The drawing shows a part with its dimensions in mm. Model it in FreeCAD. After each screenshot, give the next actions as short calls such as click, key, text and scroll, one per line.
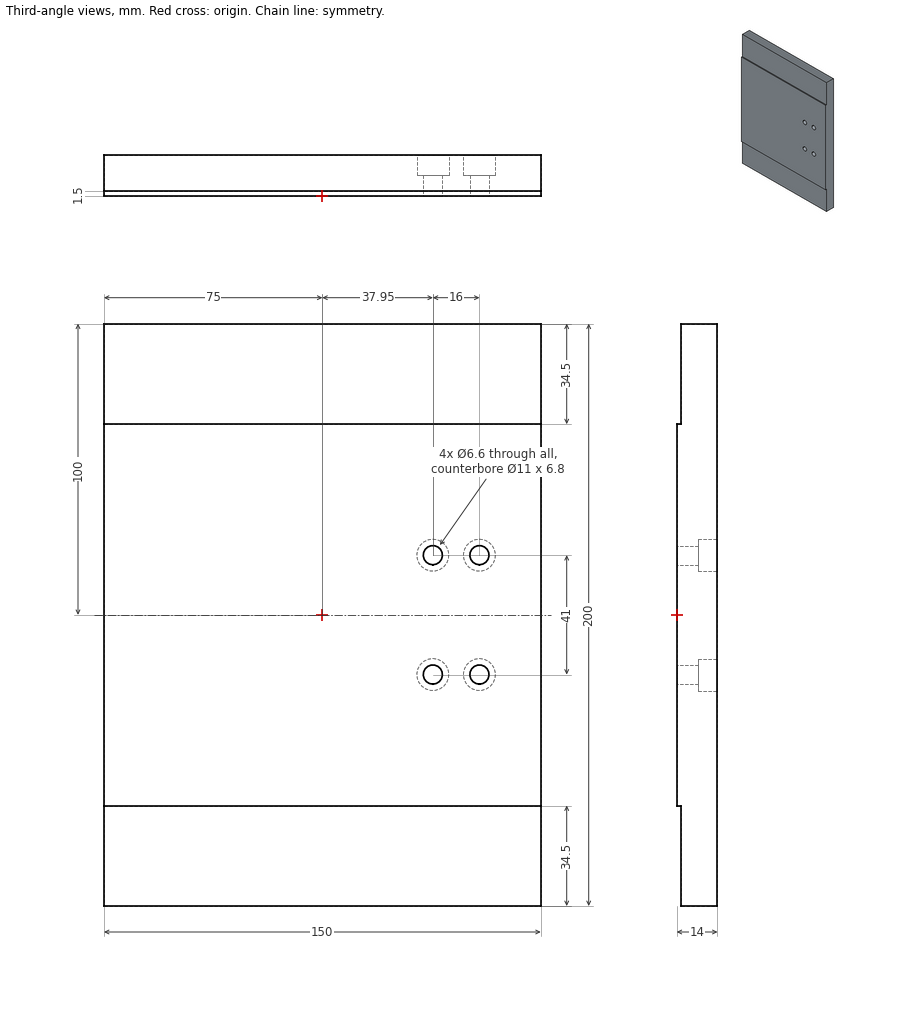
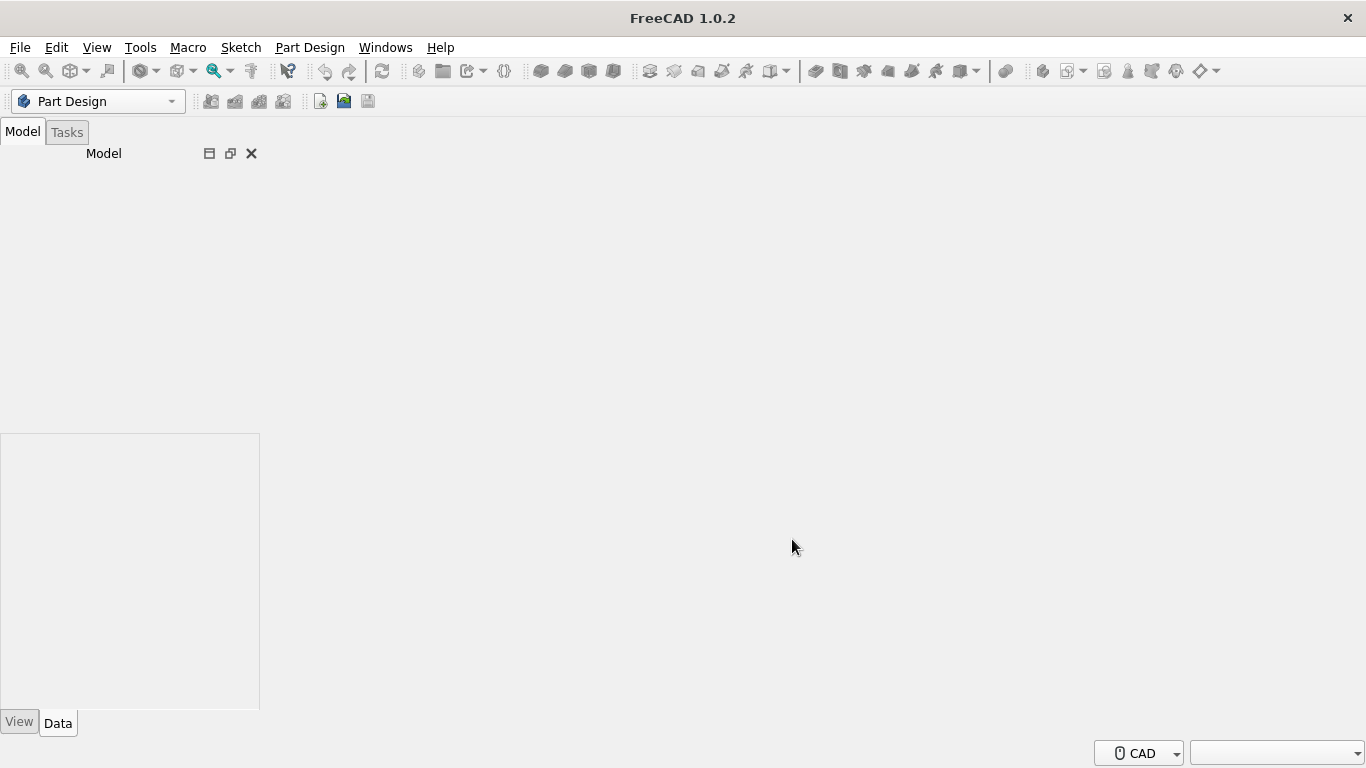
key(ctrl+n)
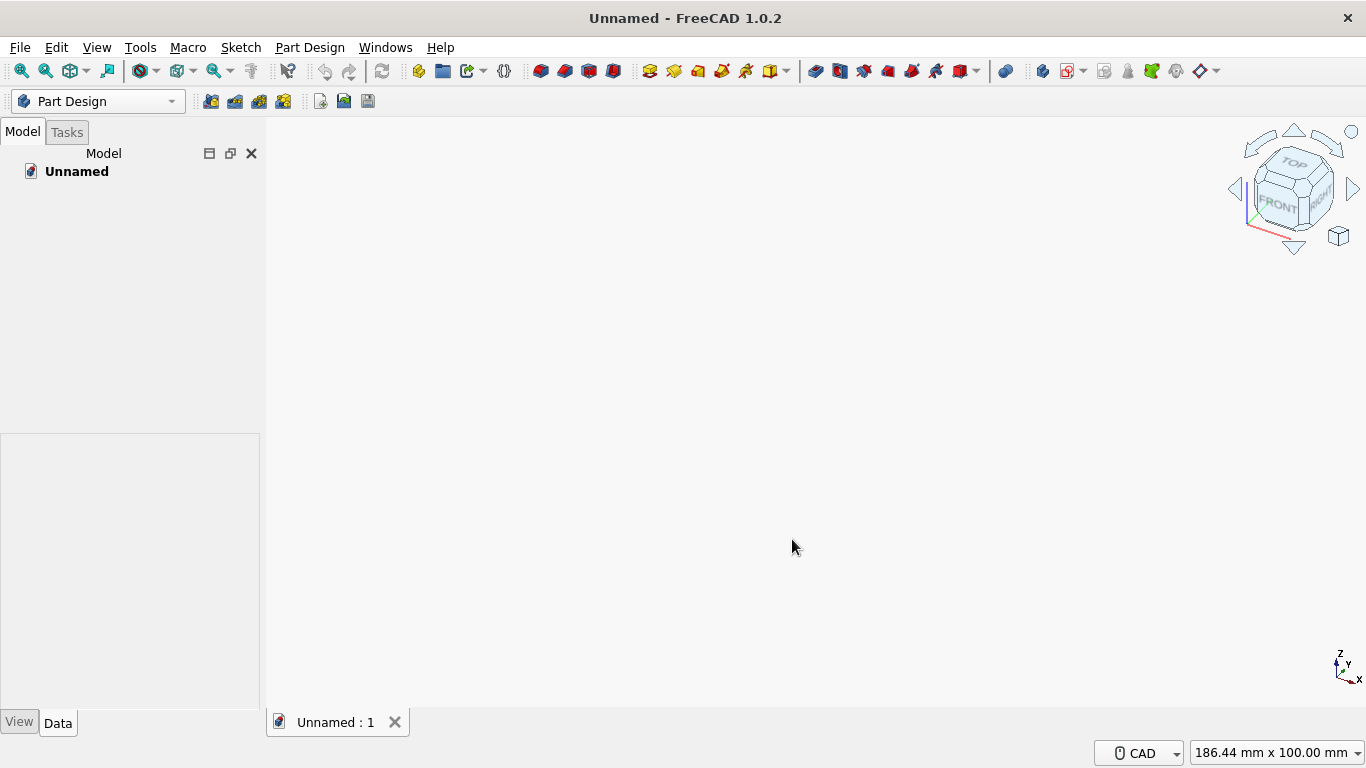
click(1068, 72)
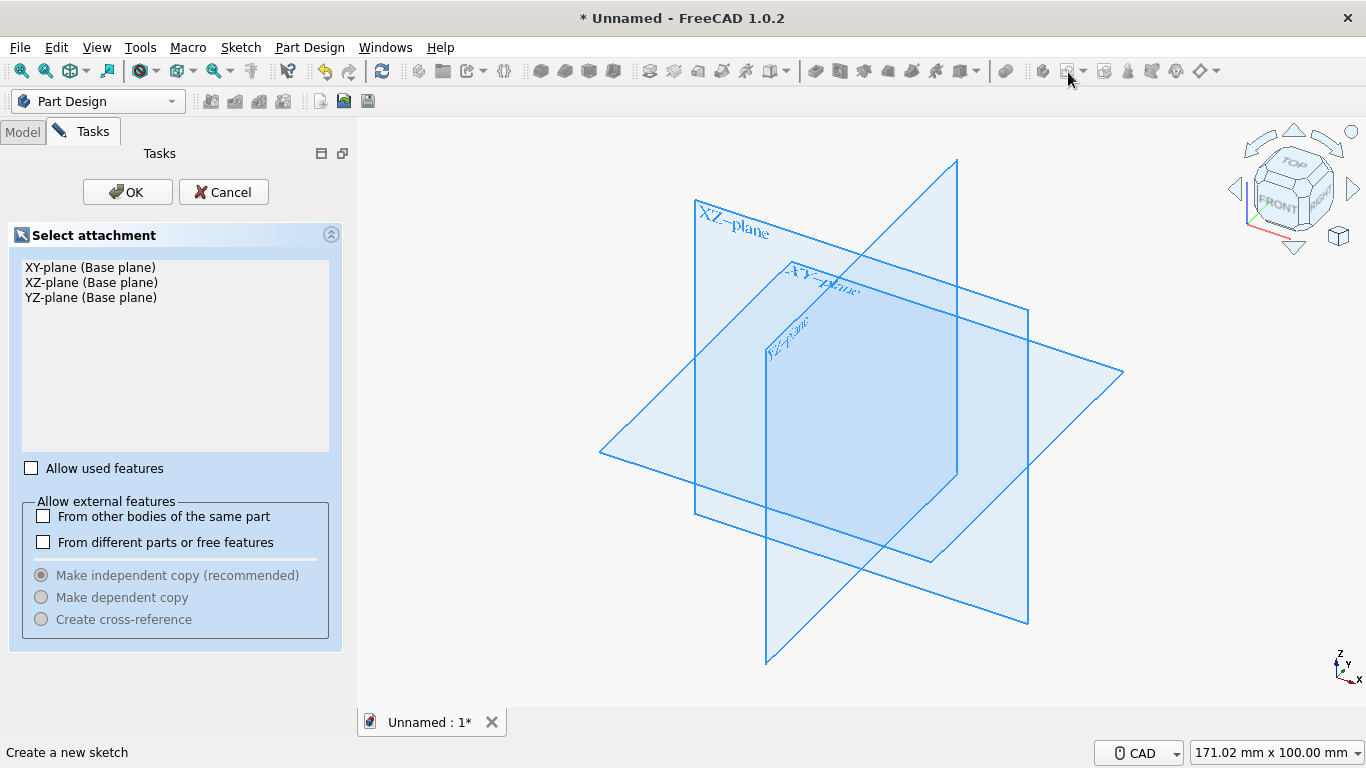
click(82, 282)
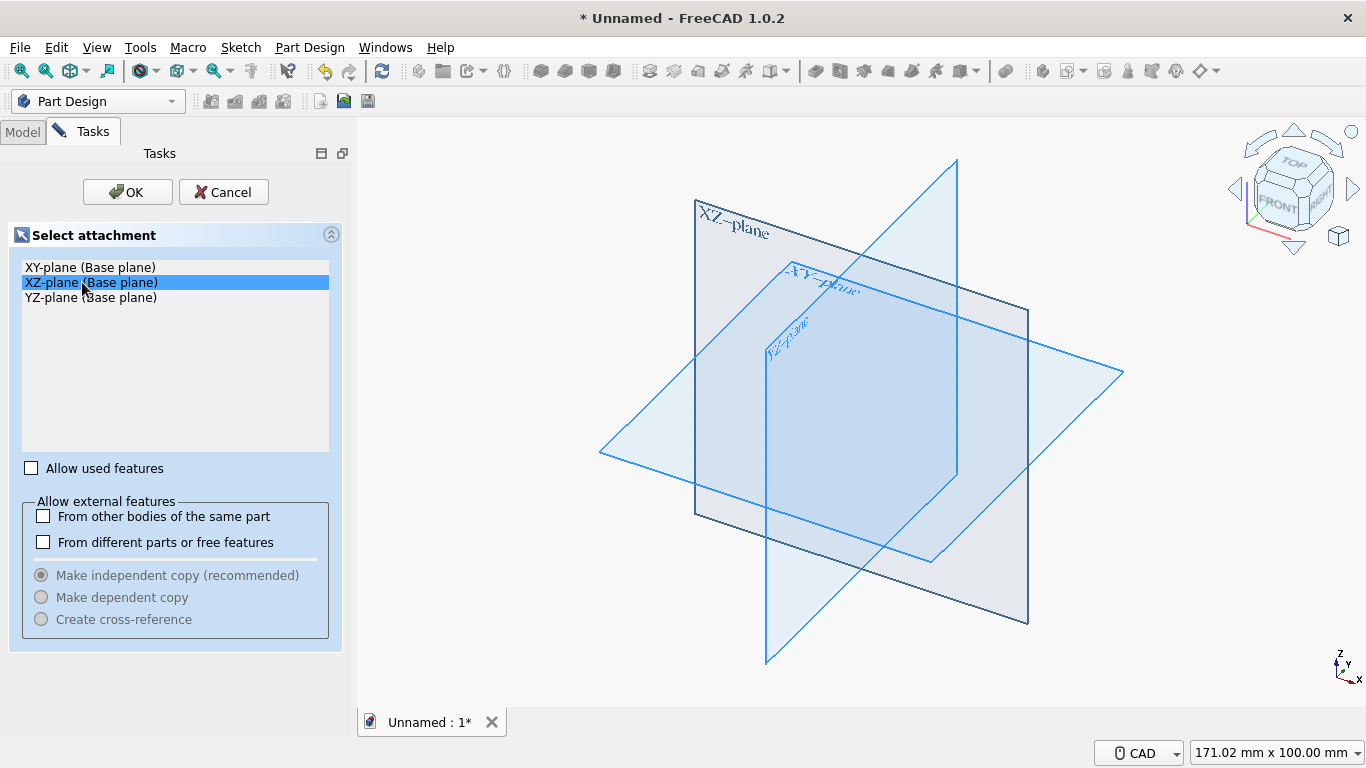
click(128, 192)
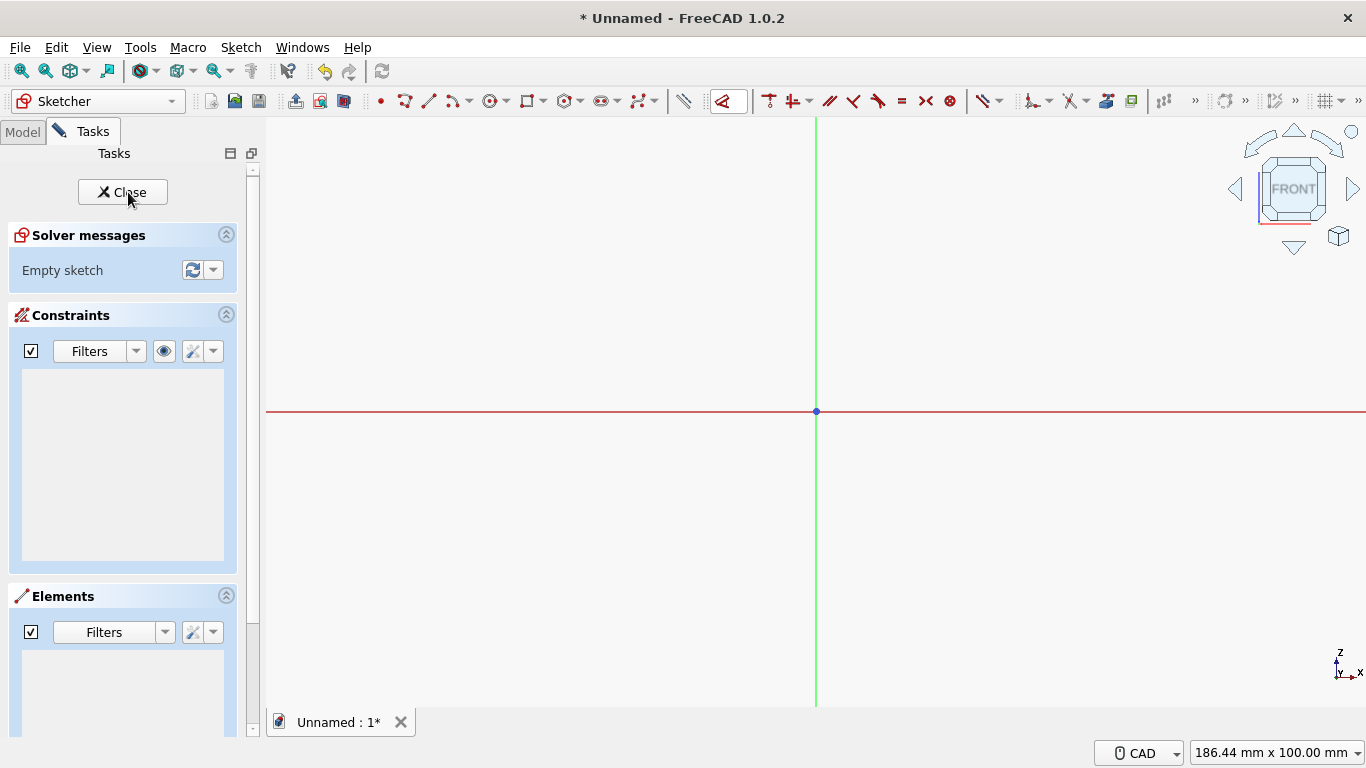
scroll(718, 412, down, 6)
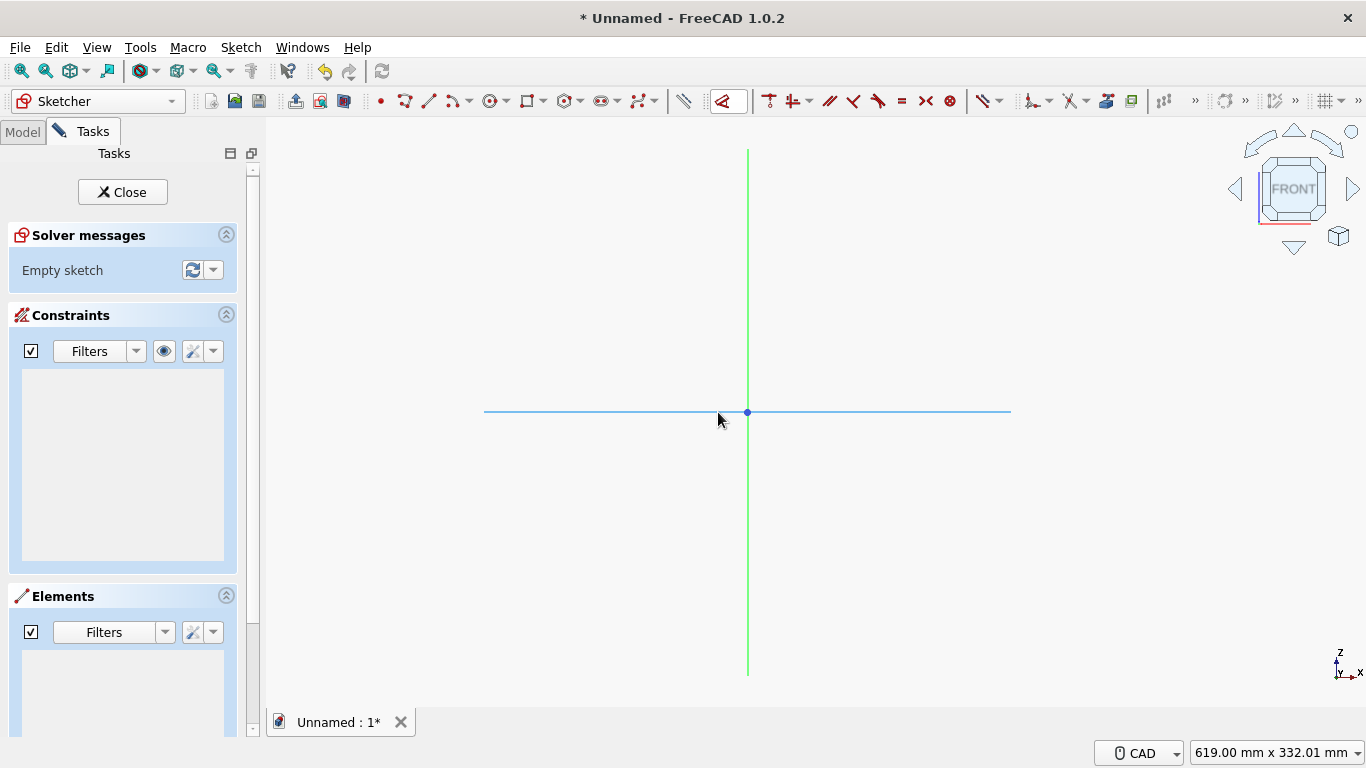
key(g)
key(v)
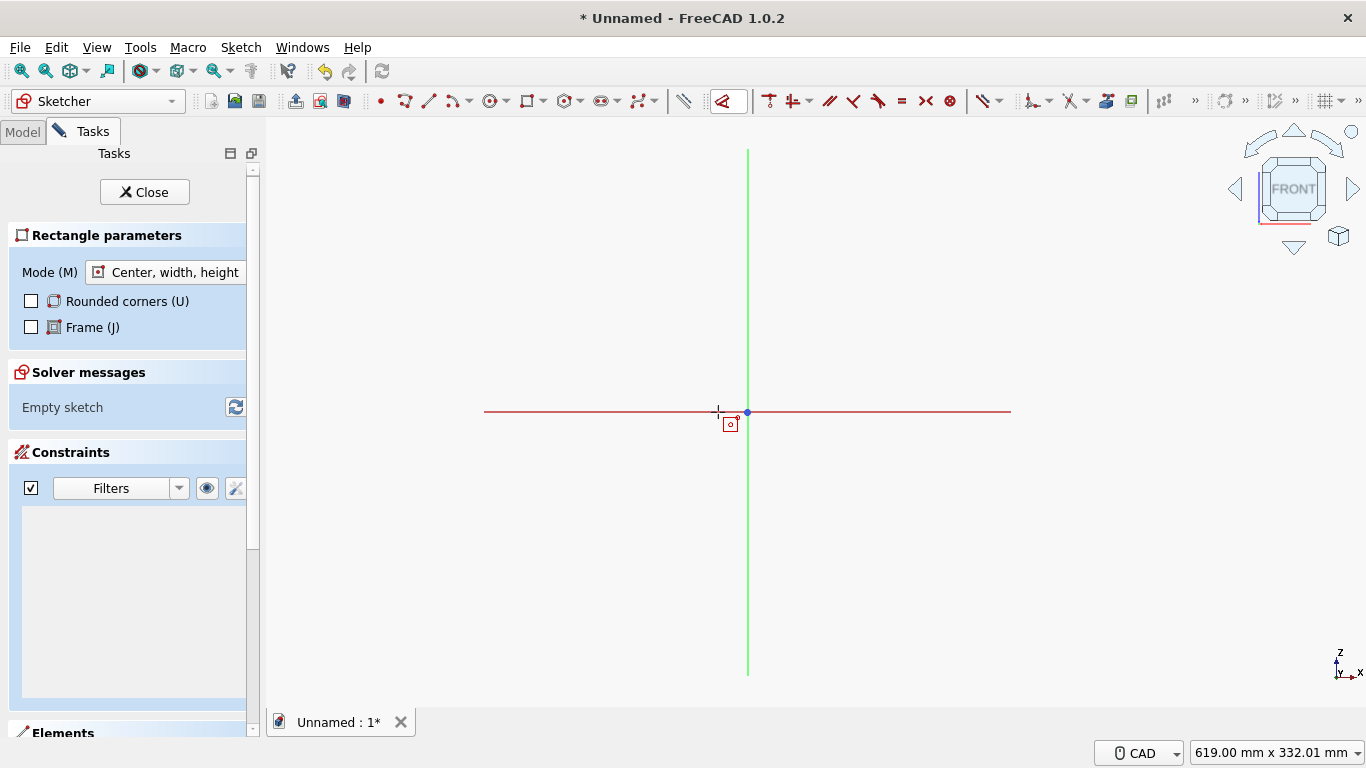
click(748, 412)
move(881, 235)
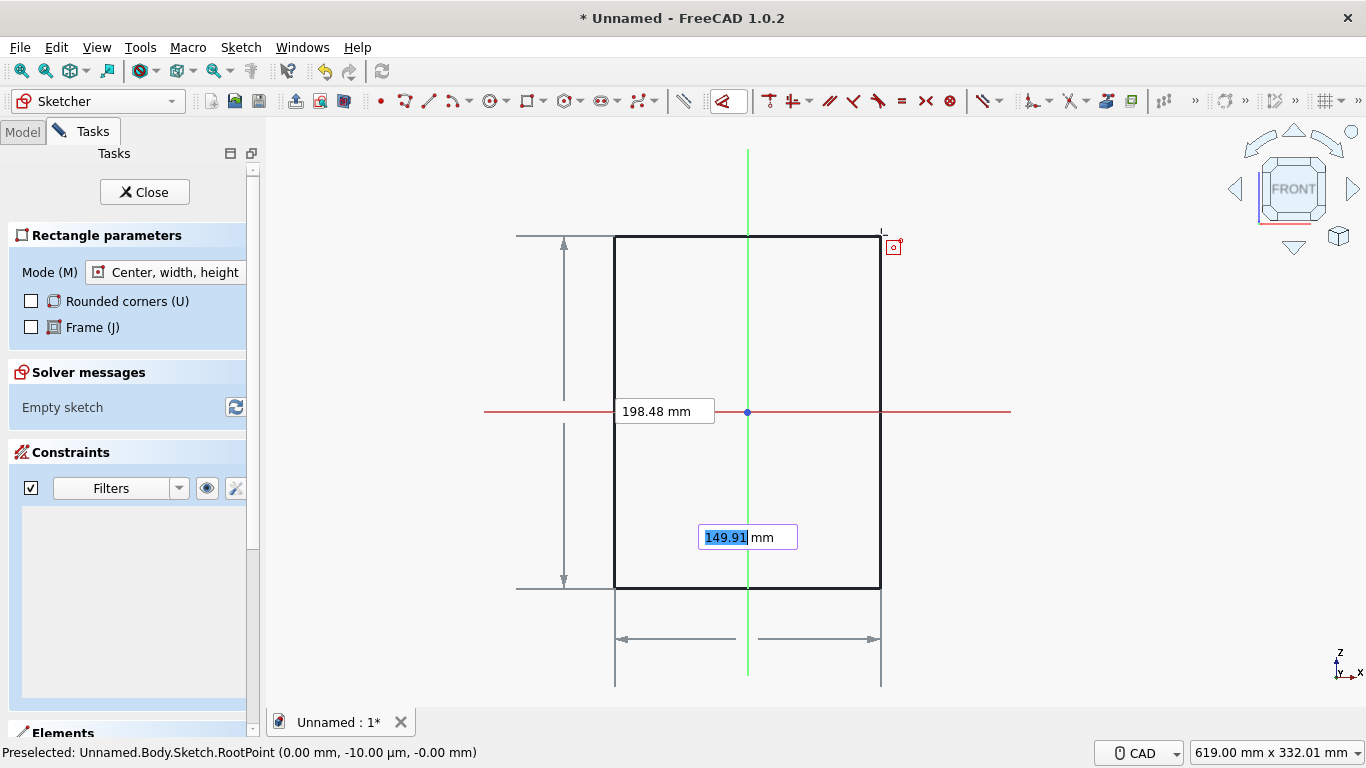
text(150)
key(Tab)
text(200)
key(Return)
key(Escape)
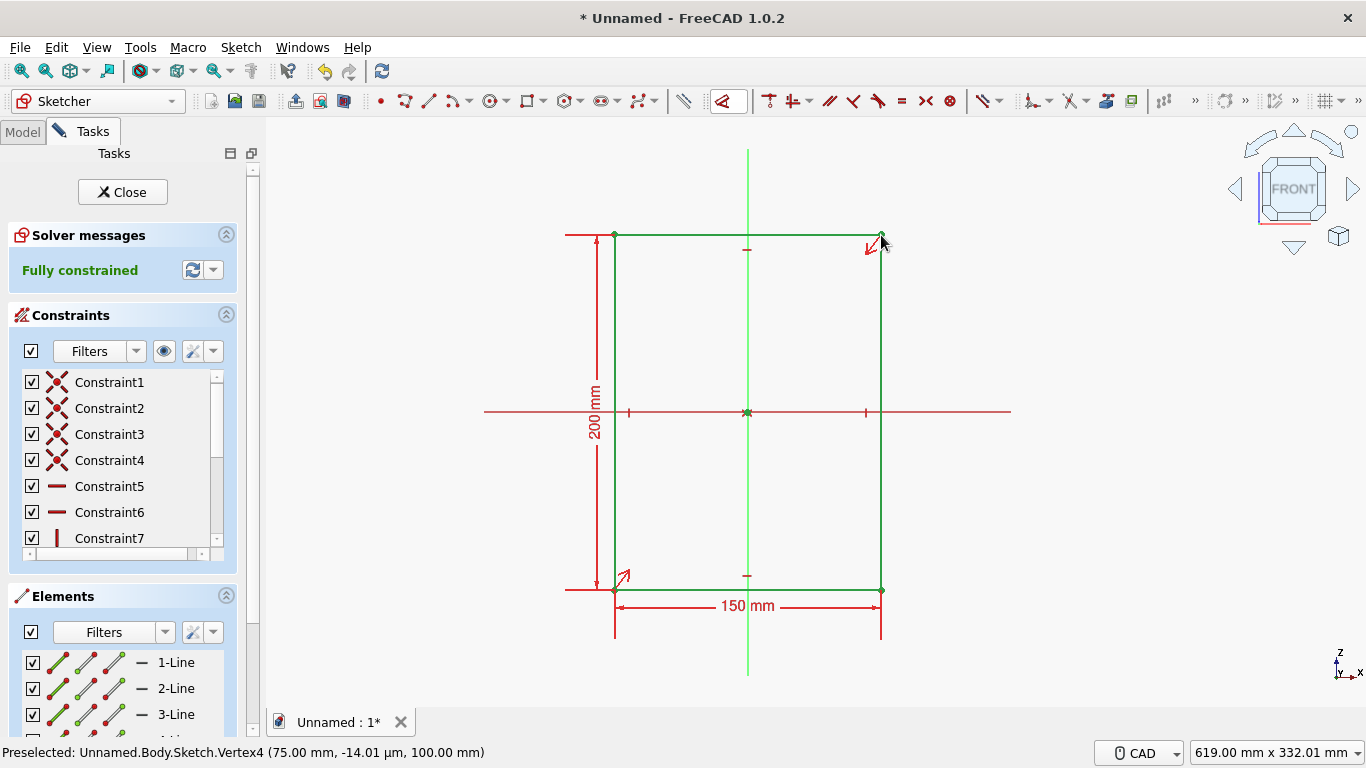
click(123, 192)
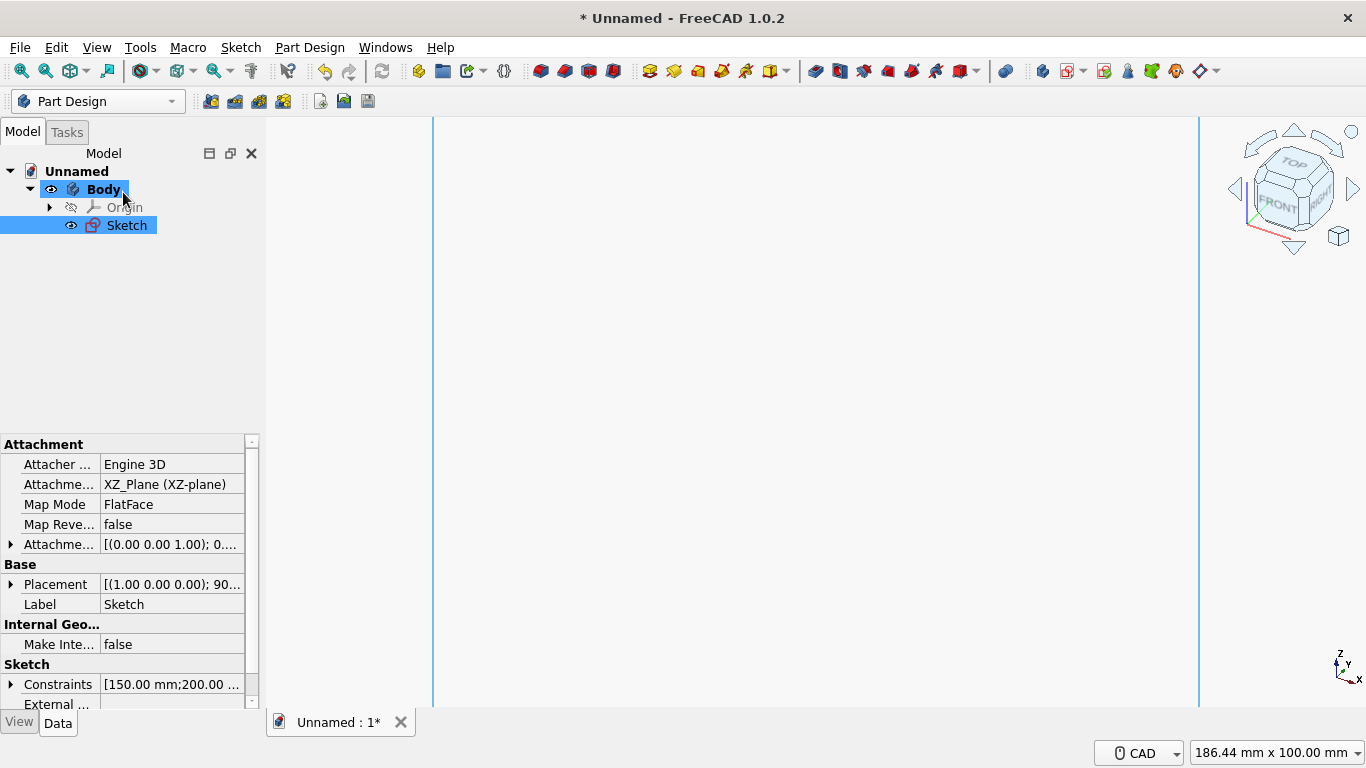
click(650, 72)